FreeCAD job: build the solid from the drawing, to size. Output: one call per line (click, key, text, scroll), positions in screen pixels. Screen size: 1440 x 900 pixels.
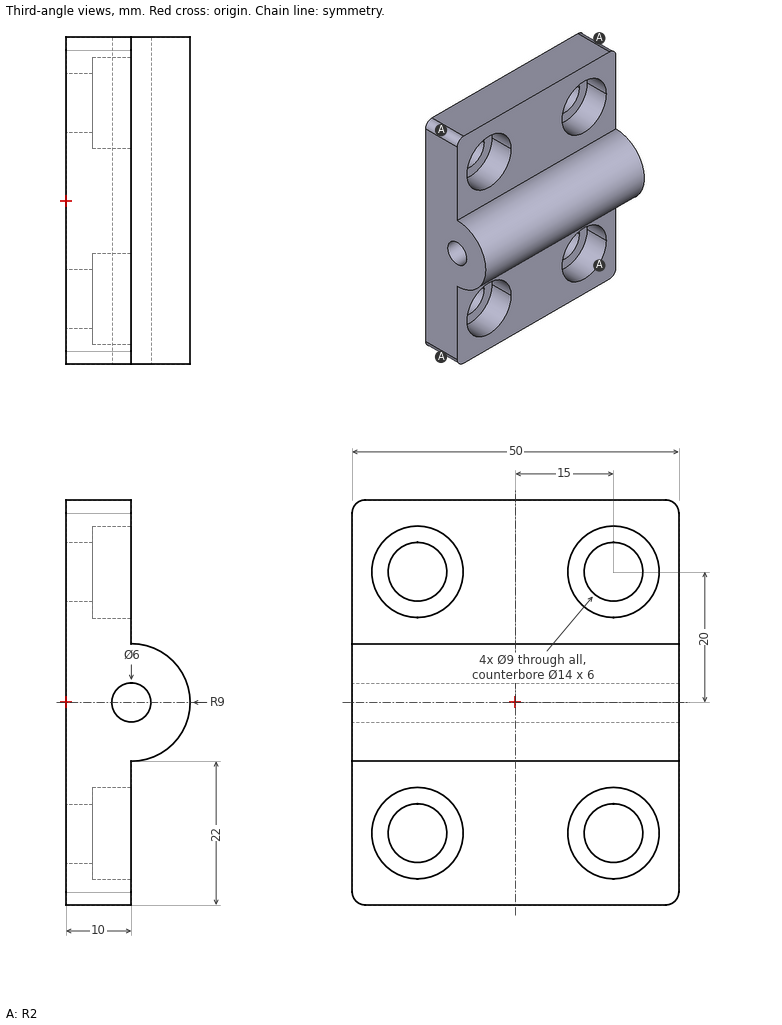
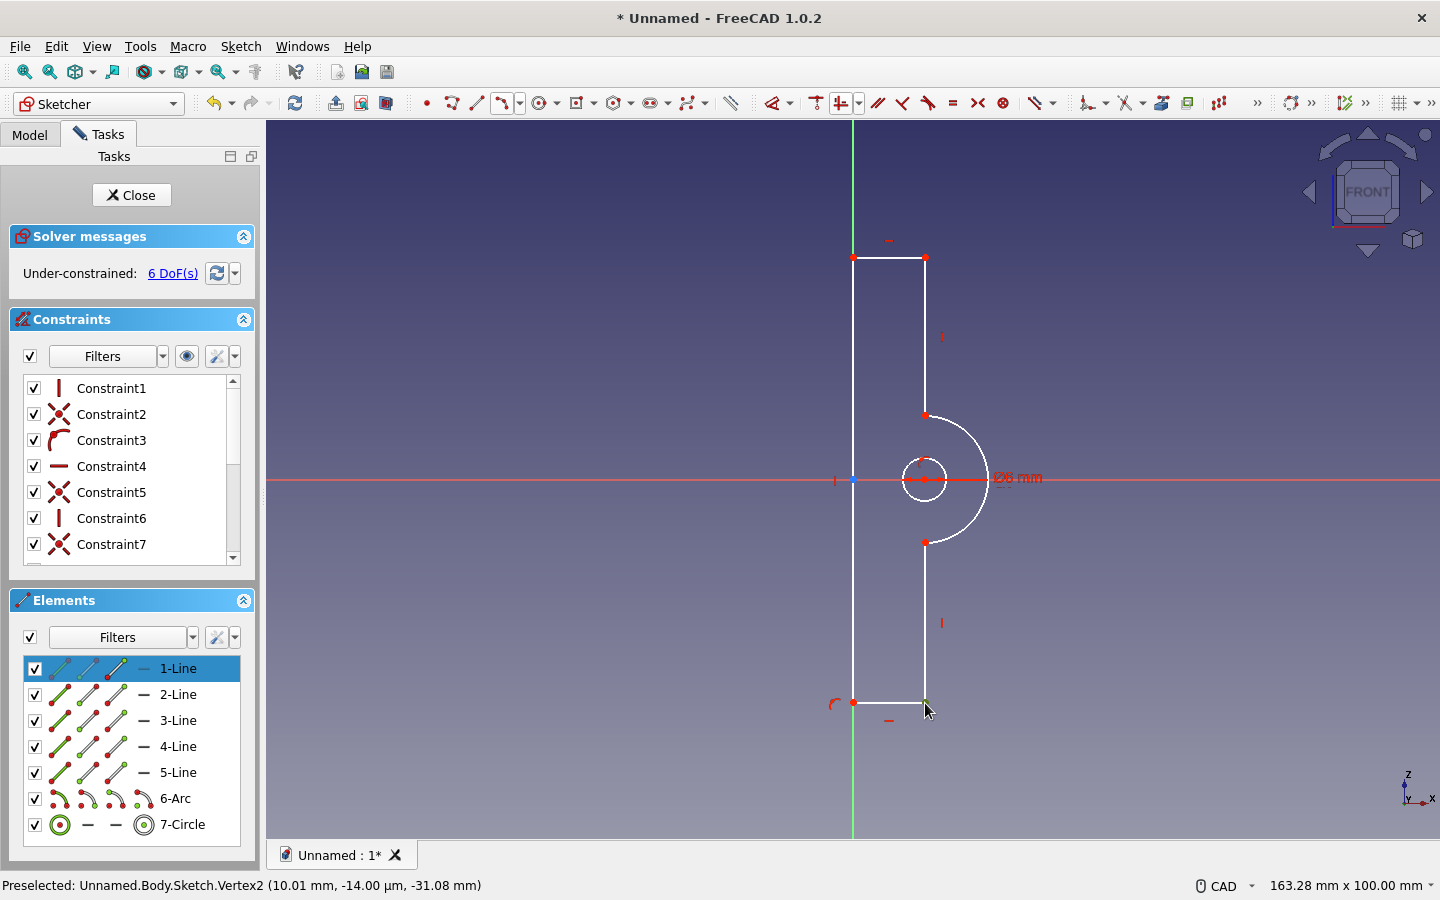
click(925, 258)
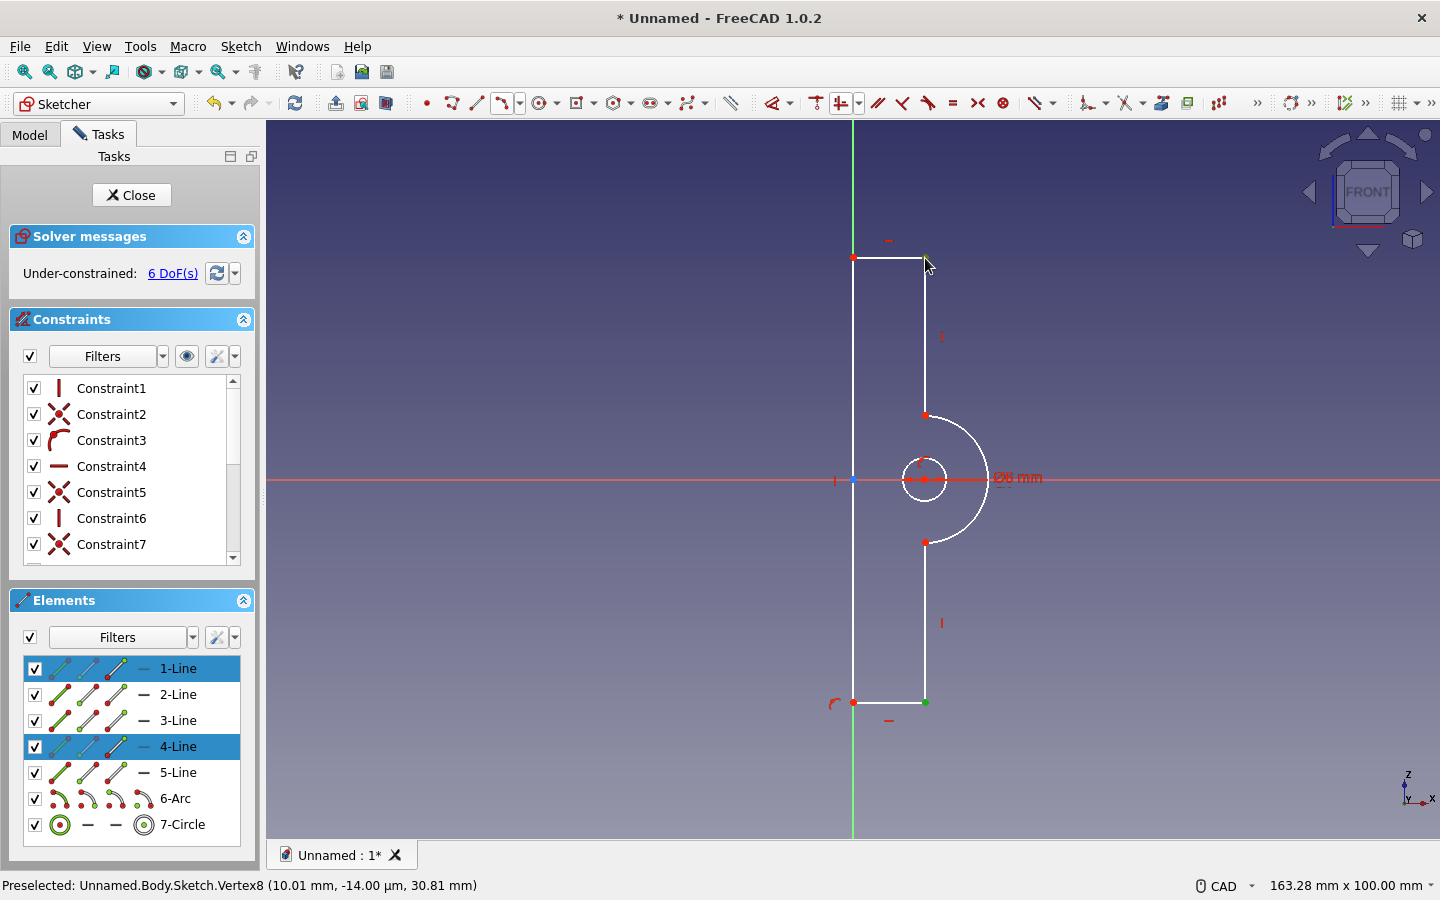
click(364, 480)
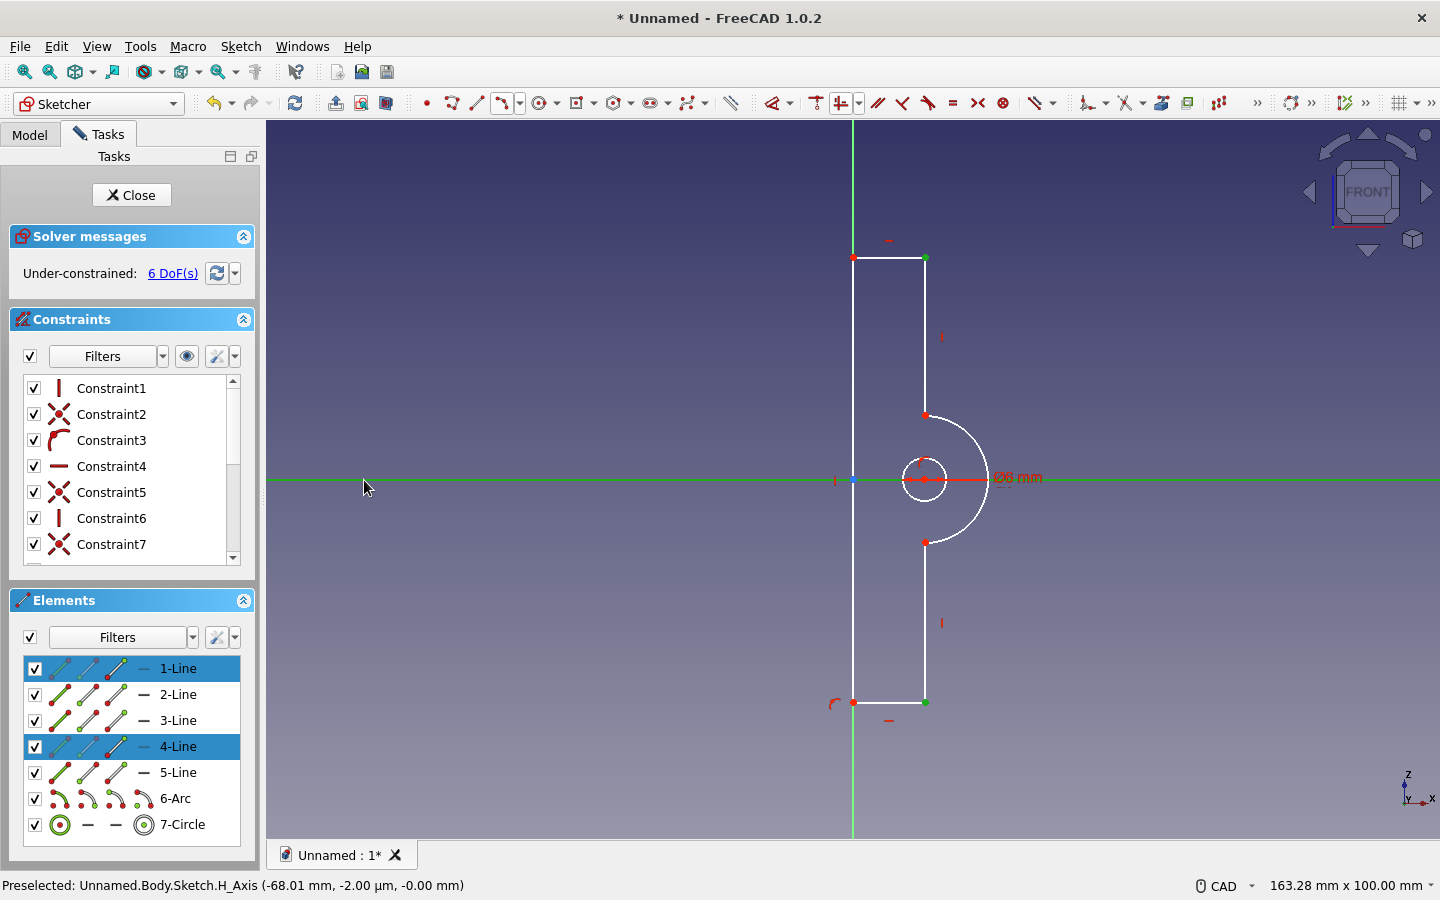
click(978, 104)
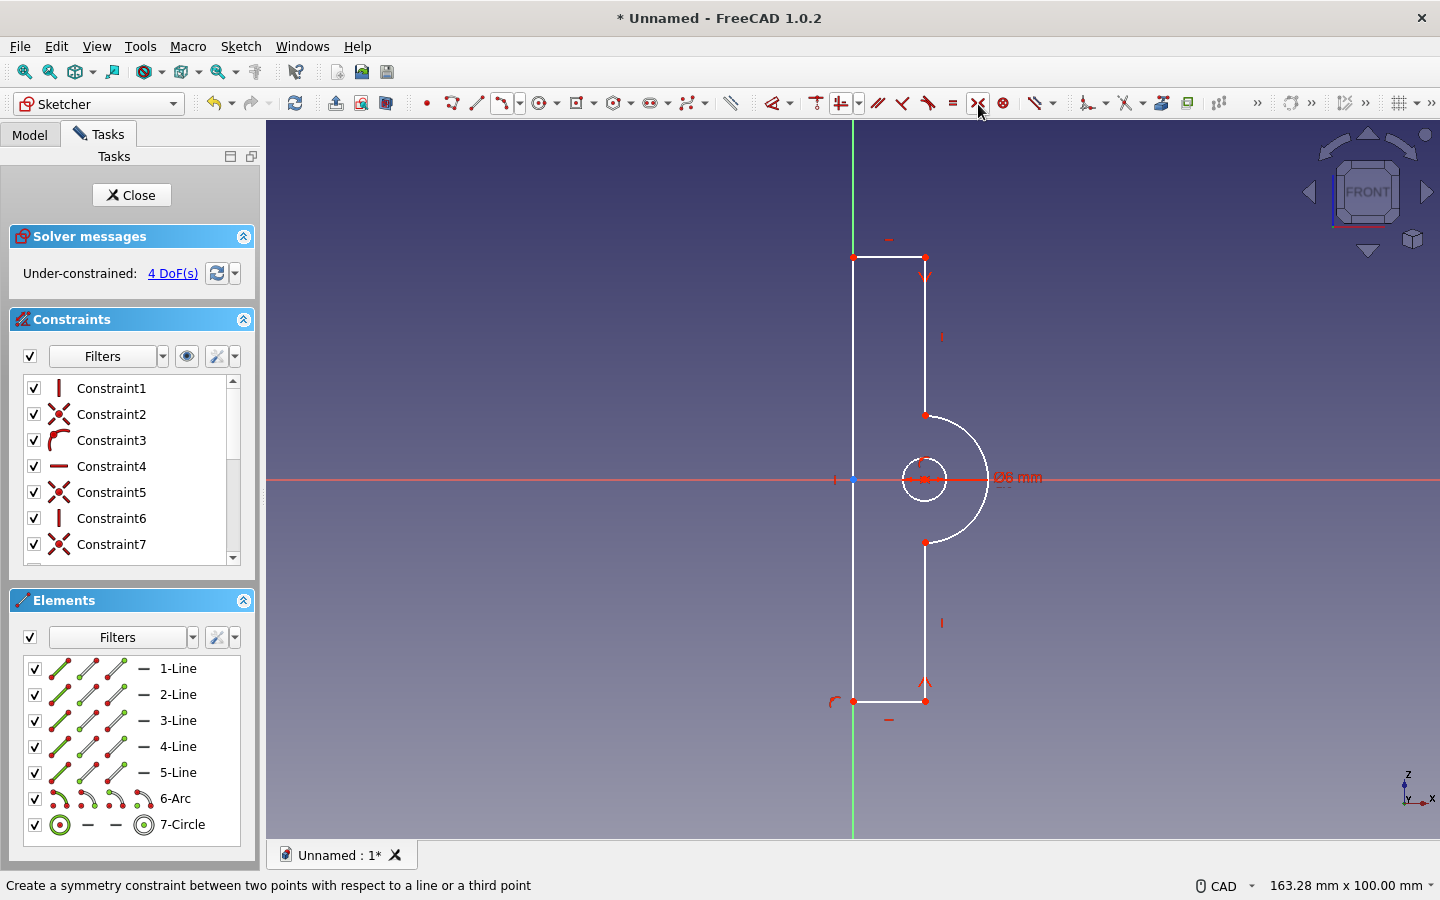
click(772, 104)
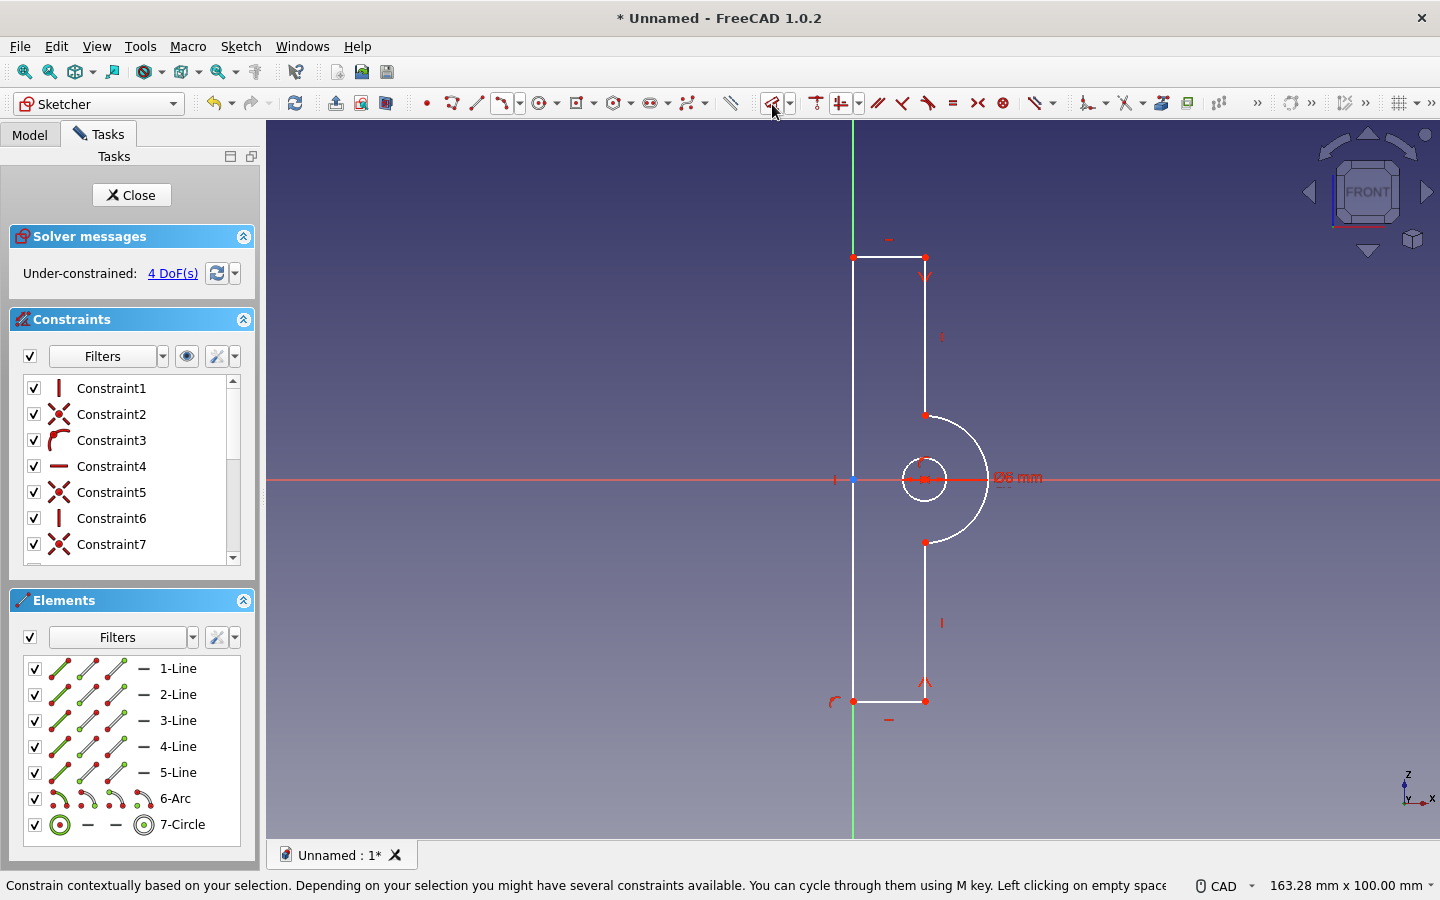
click(976, 517)
click(1002, 536)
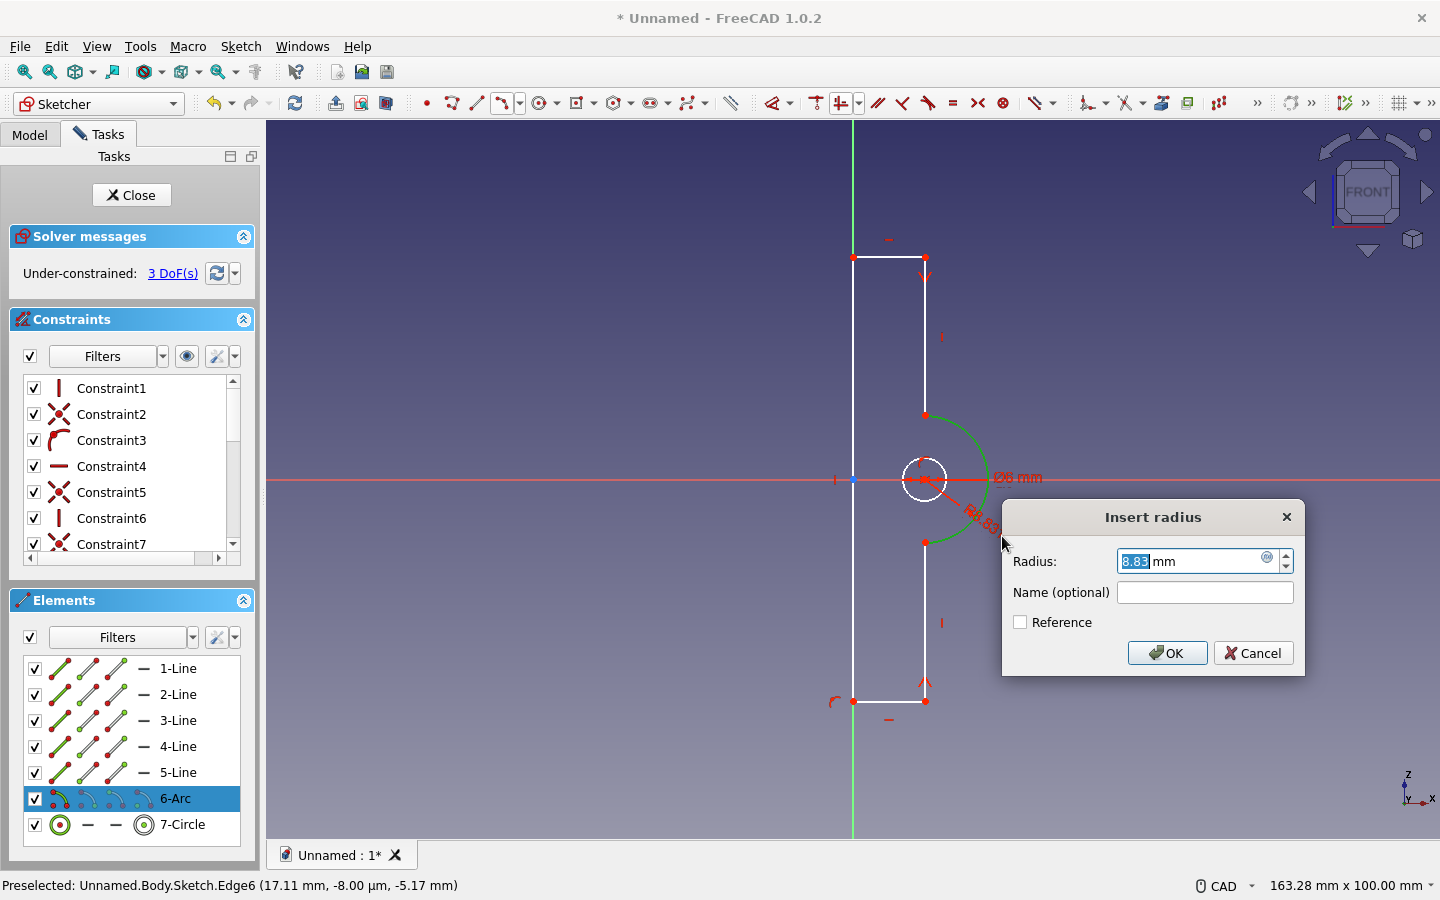
text(9)
key(Return)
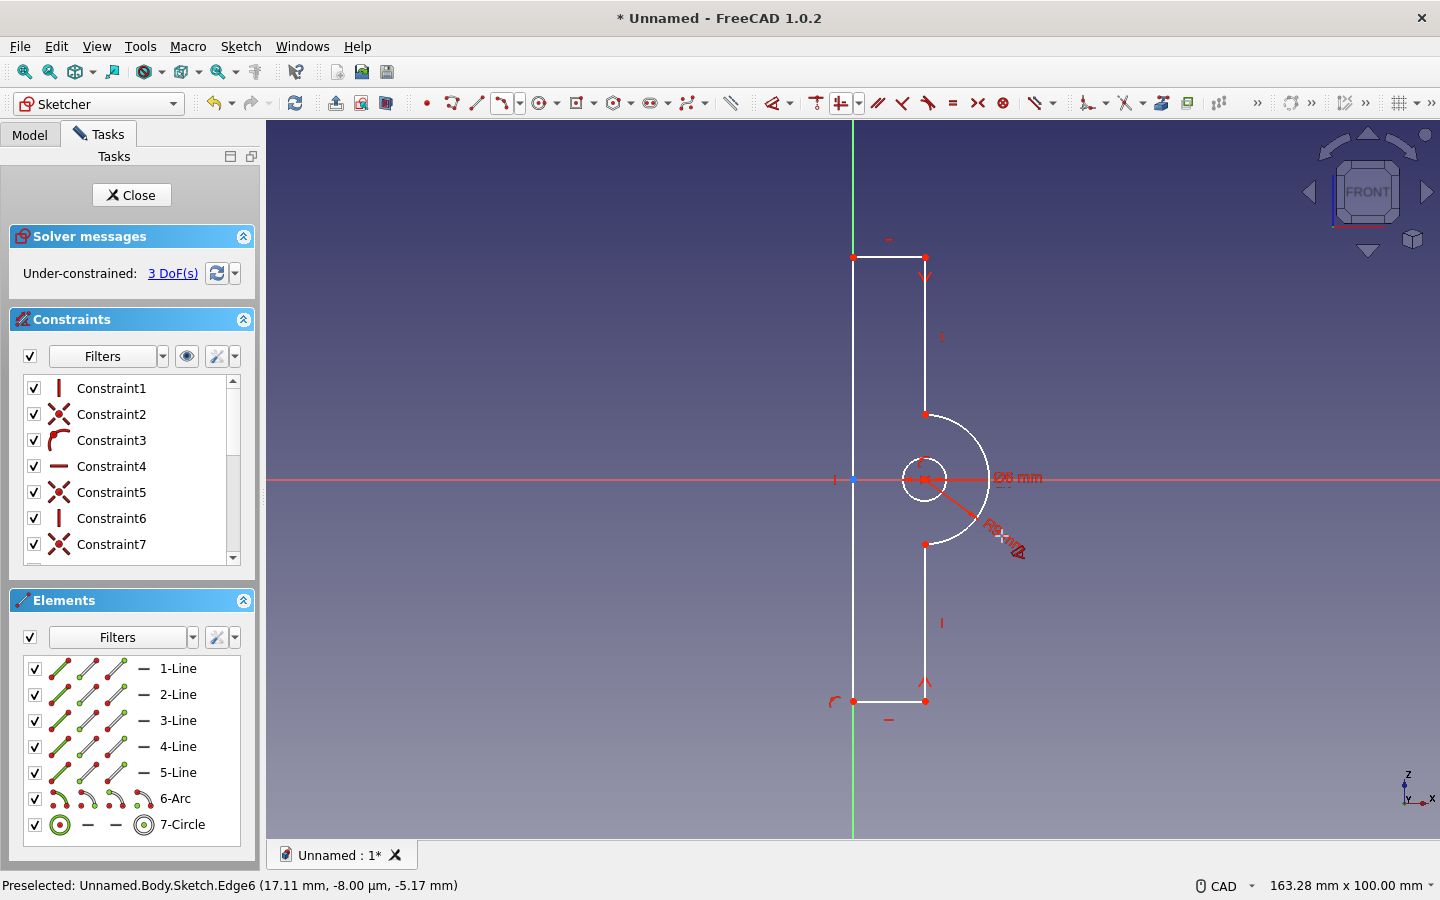
click(925, 591)
click(959, 623)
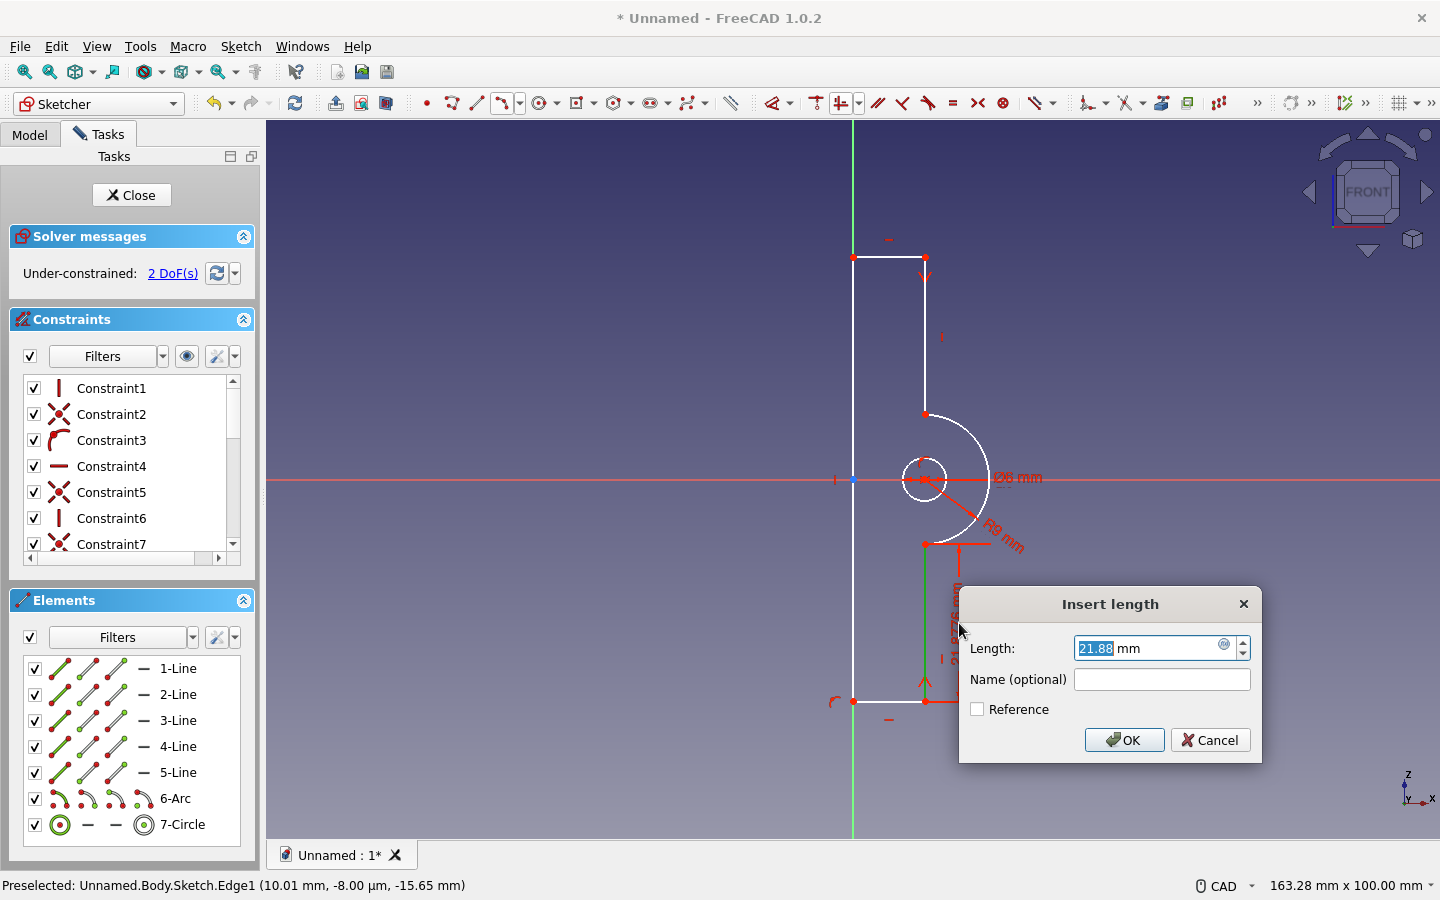
text(22)
key(Return)